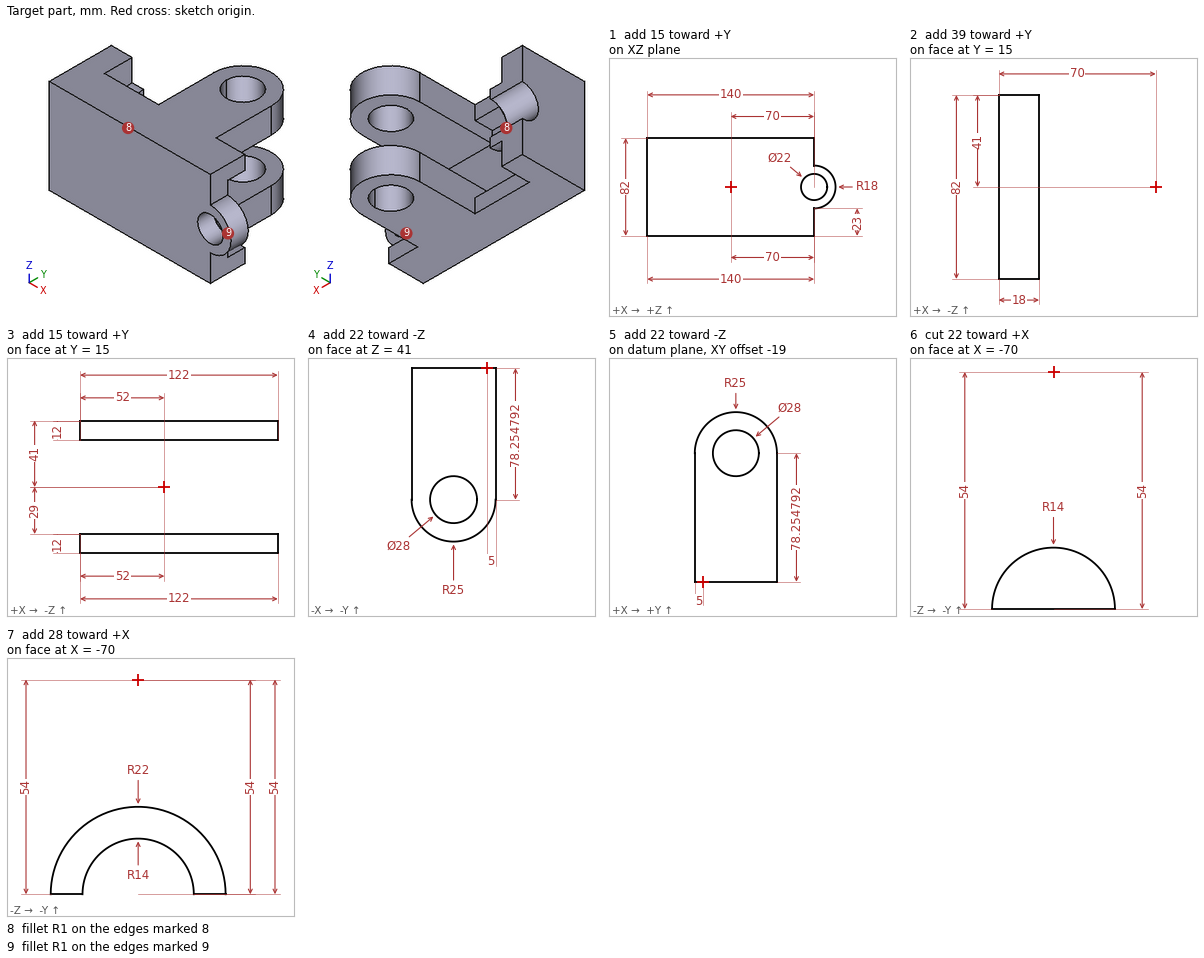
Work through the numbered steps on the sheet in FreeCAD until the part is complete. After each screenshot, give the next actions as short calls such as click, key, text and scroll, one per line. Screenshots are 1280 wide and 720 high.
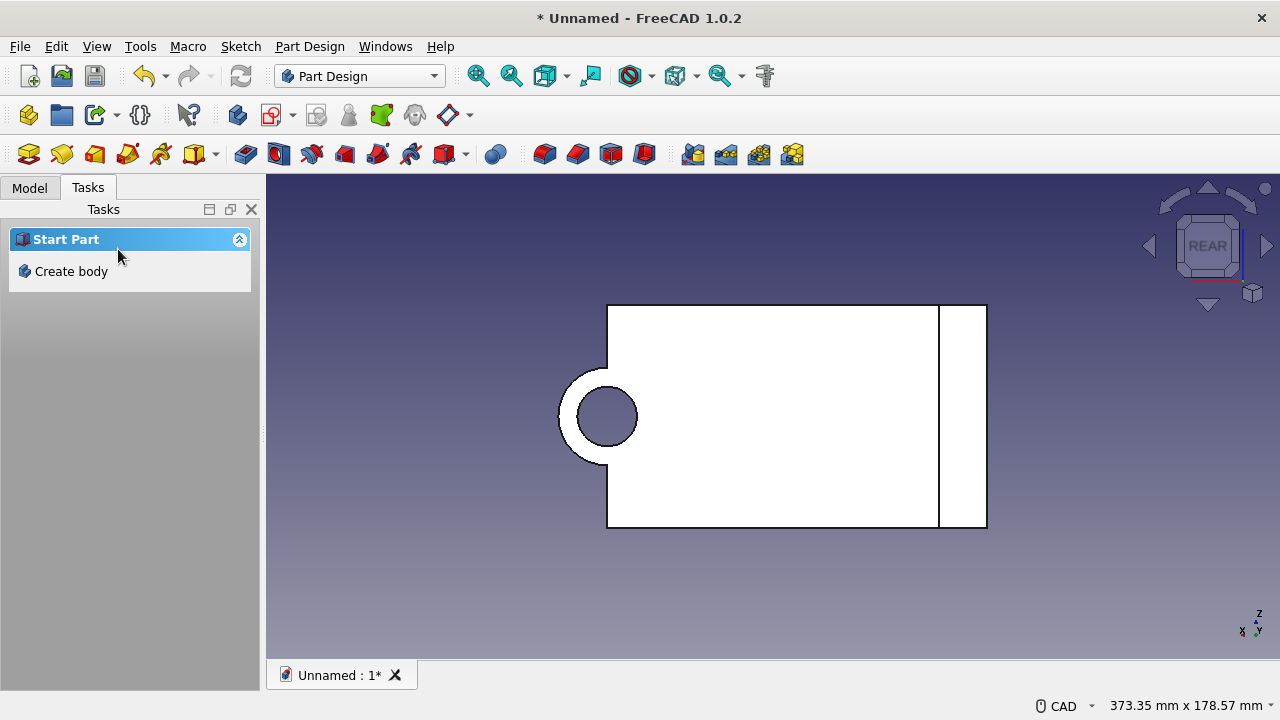
click(748, 416)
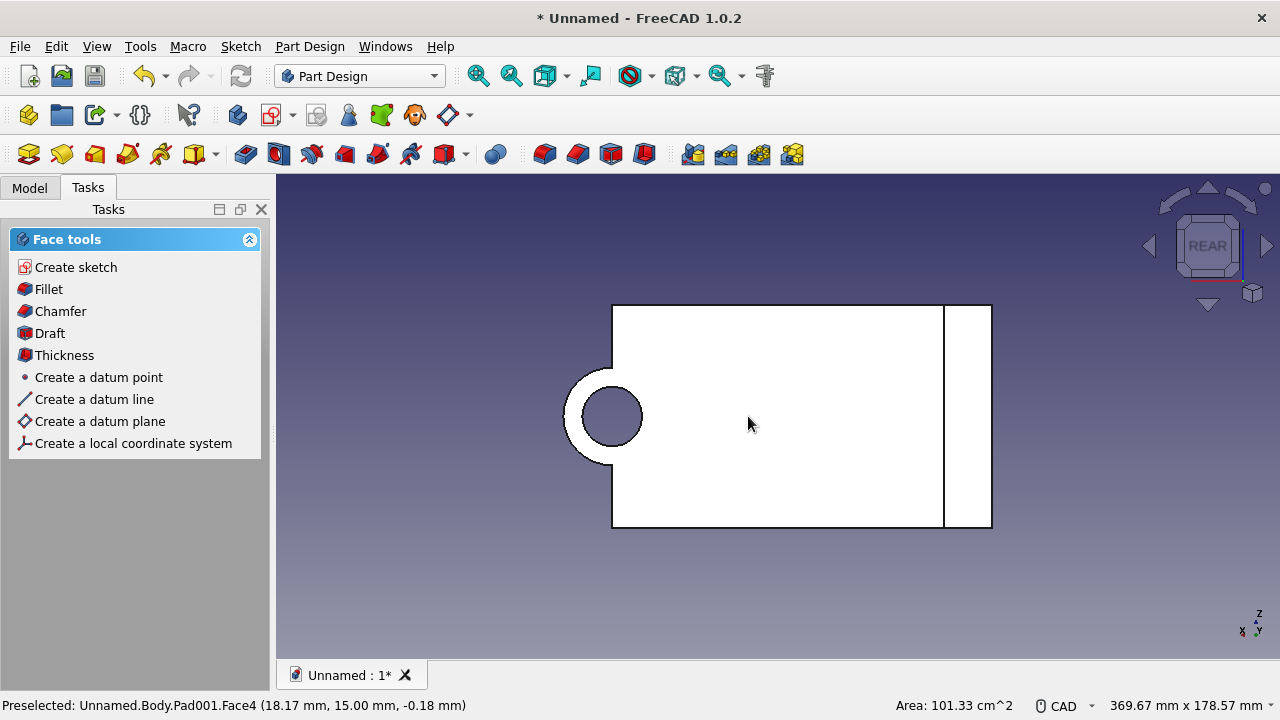
click(270, 116)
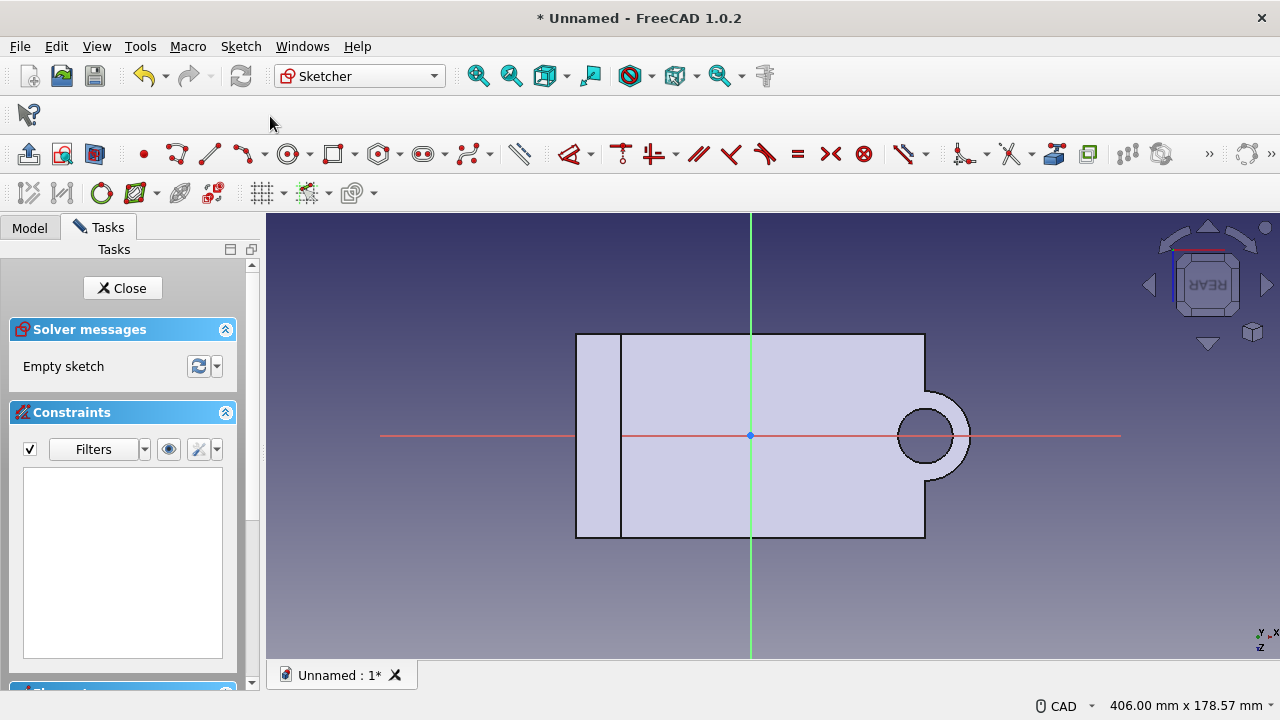
click(95, 154)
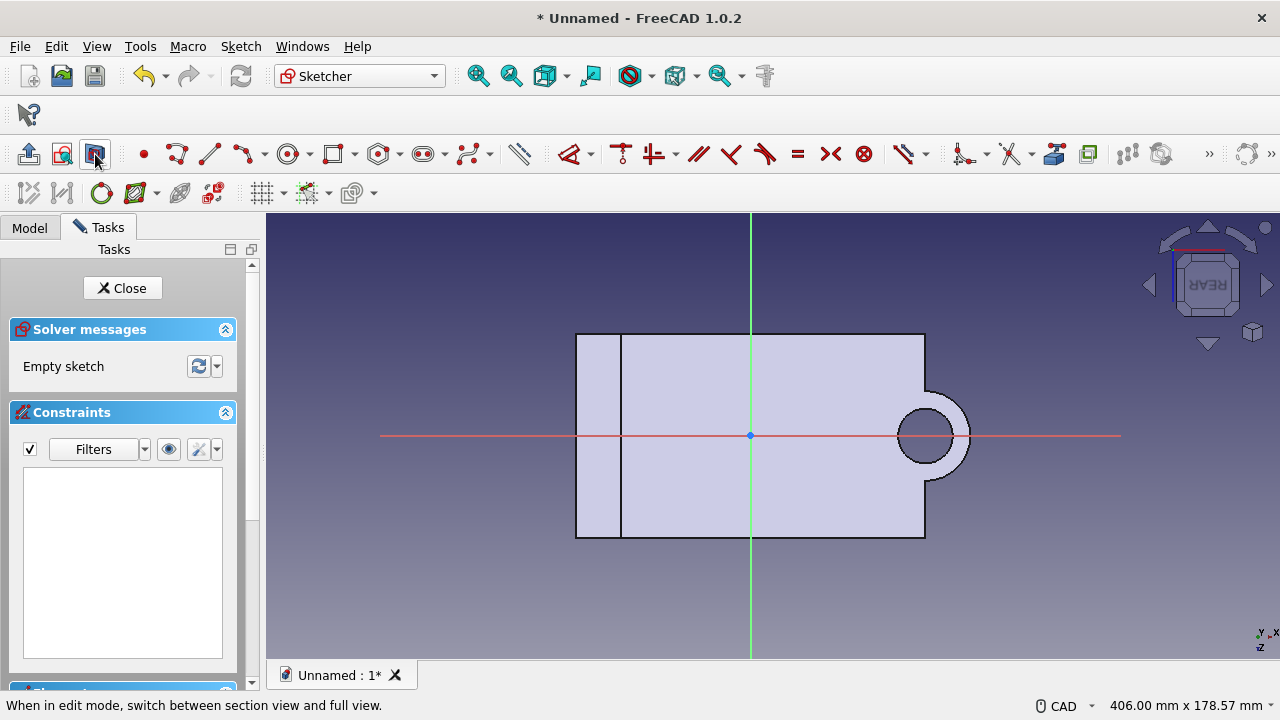
click(332, 154)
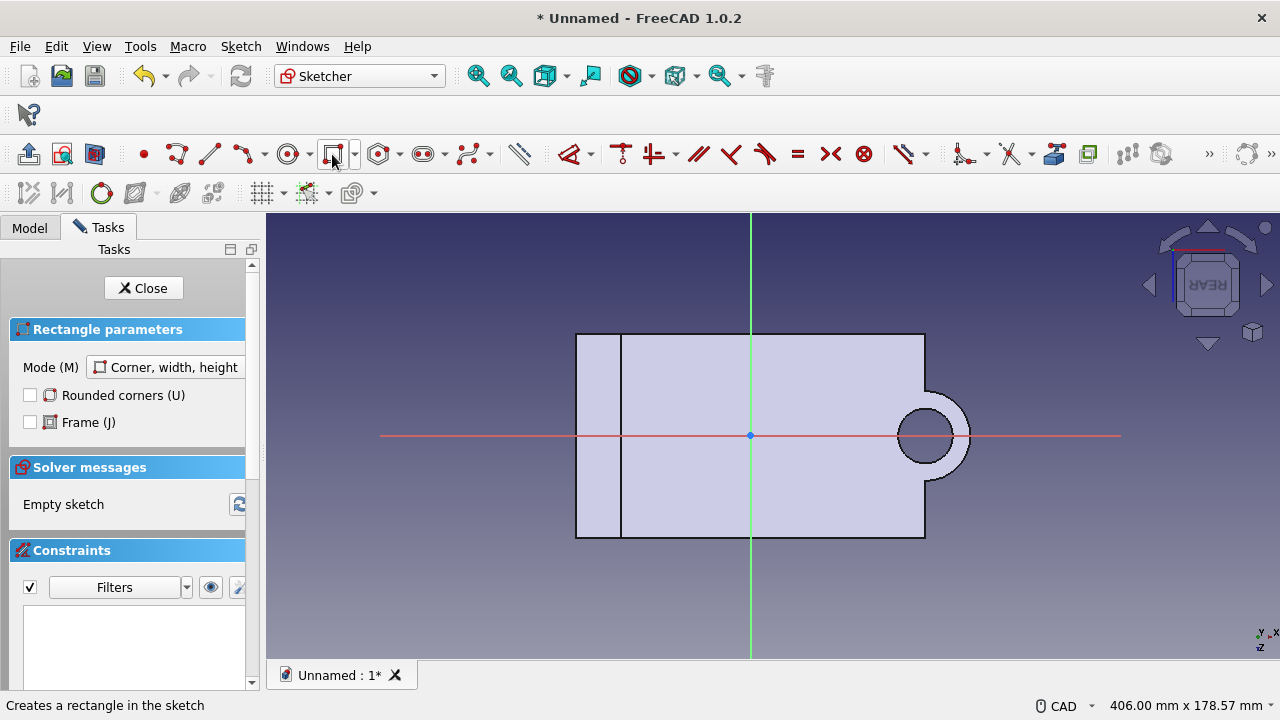
click(621, 334)
click(925, 364)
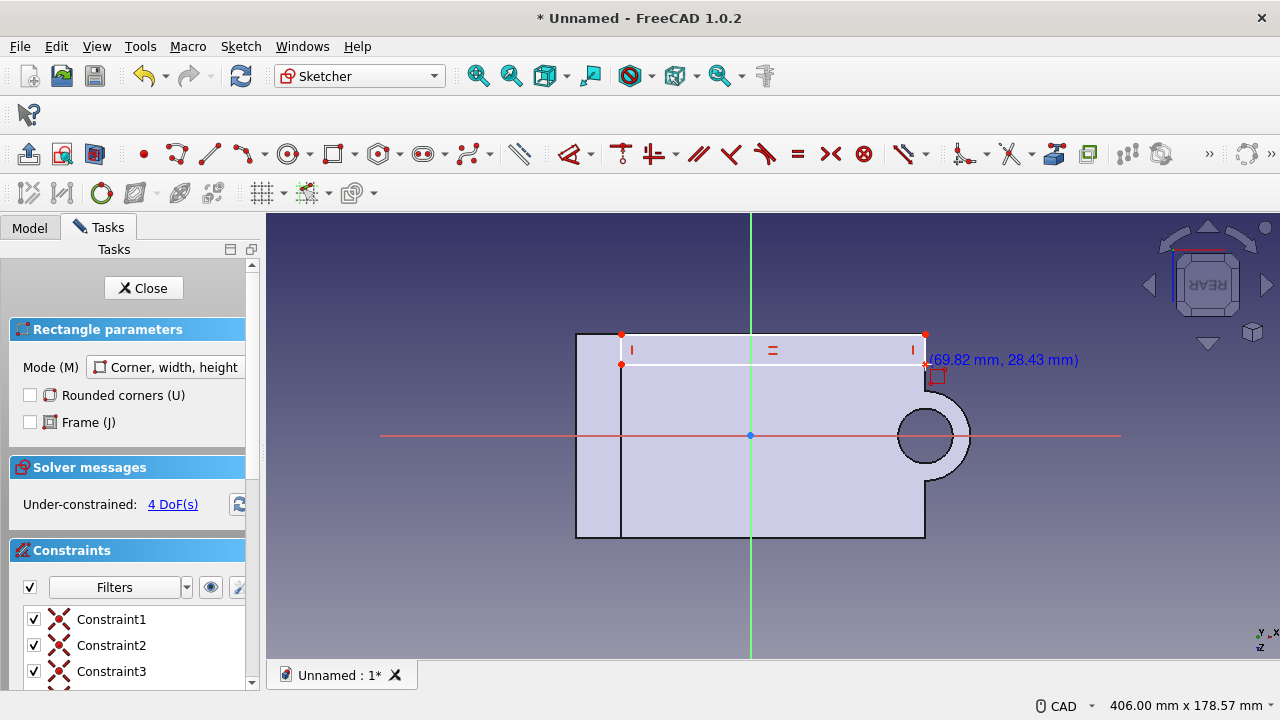
click(621, 508)
click(925, 538)
key(Escape)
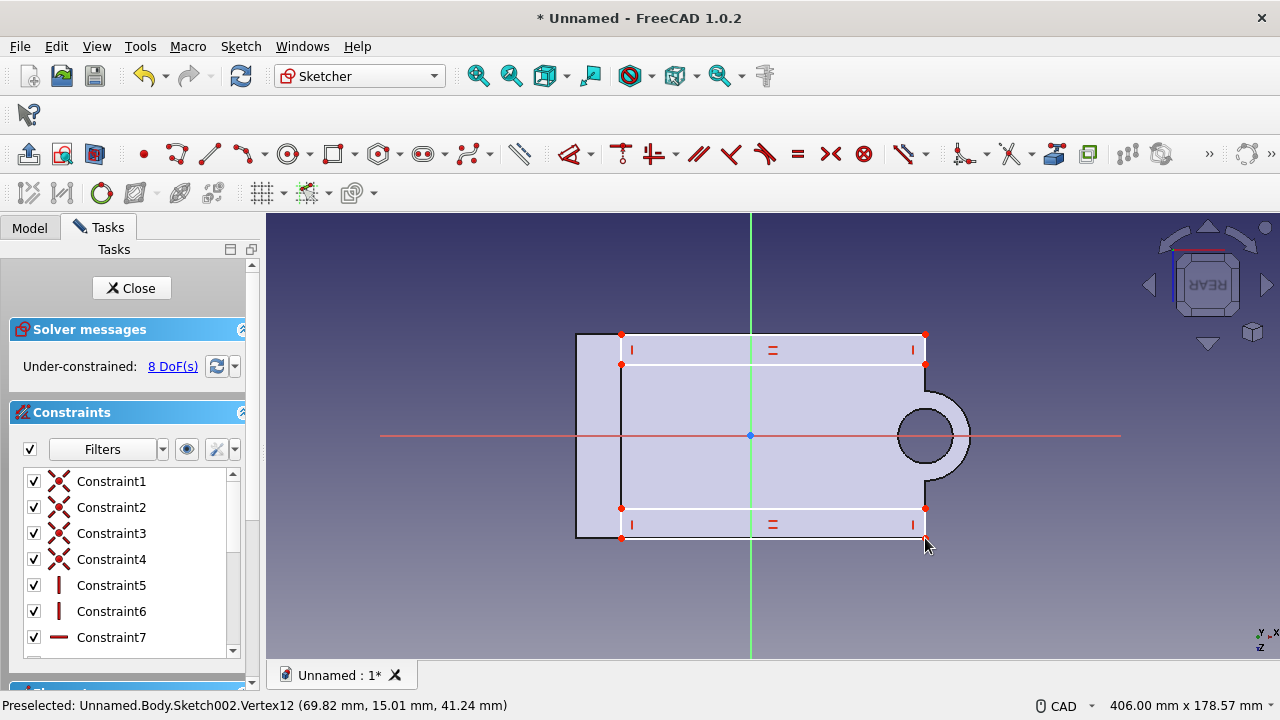
click(568, 154)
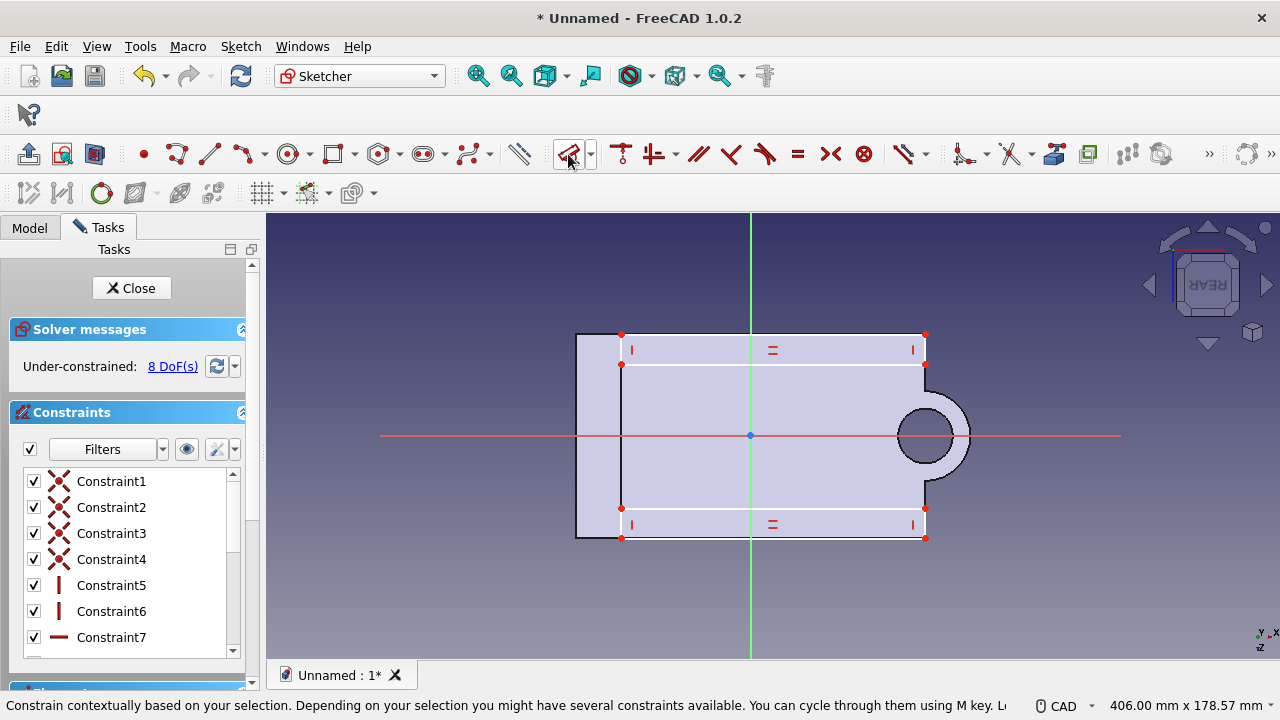
scroll(621, 344, up, 3)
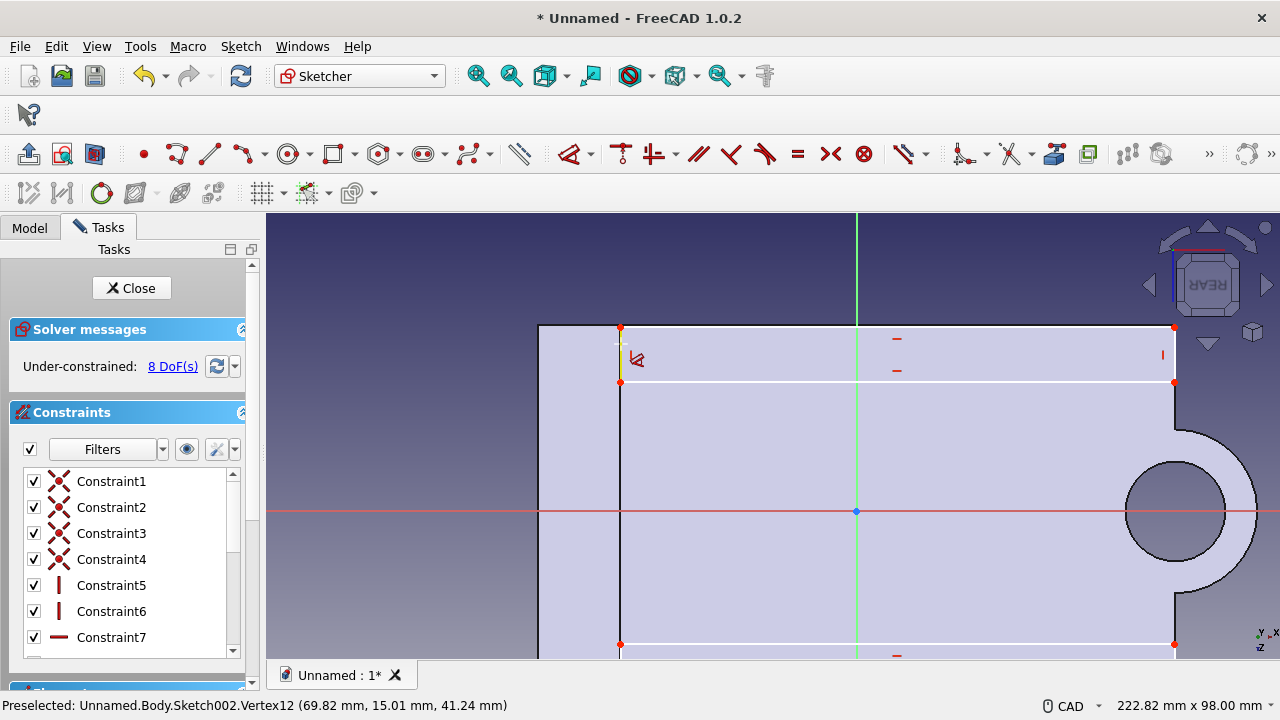
click(621, 344)
click(587, 355)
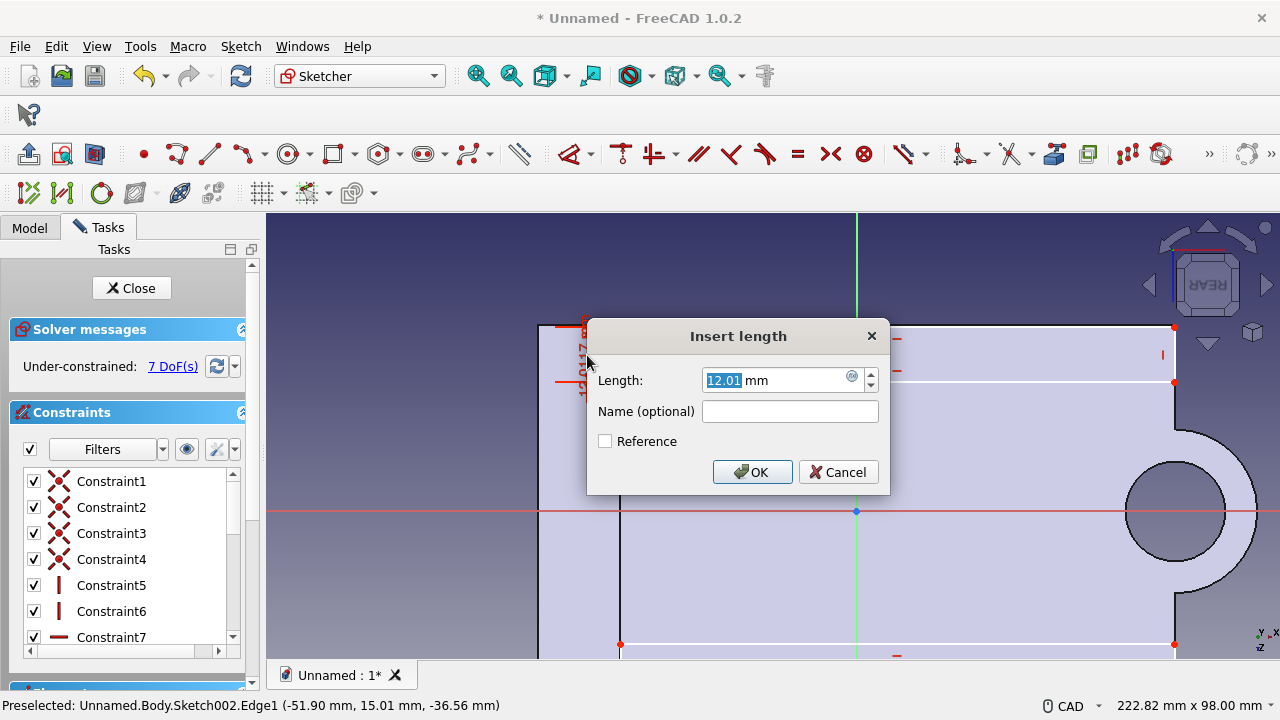
text(12)
key(Return)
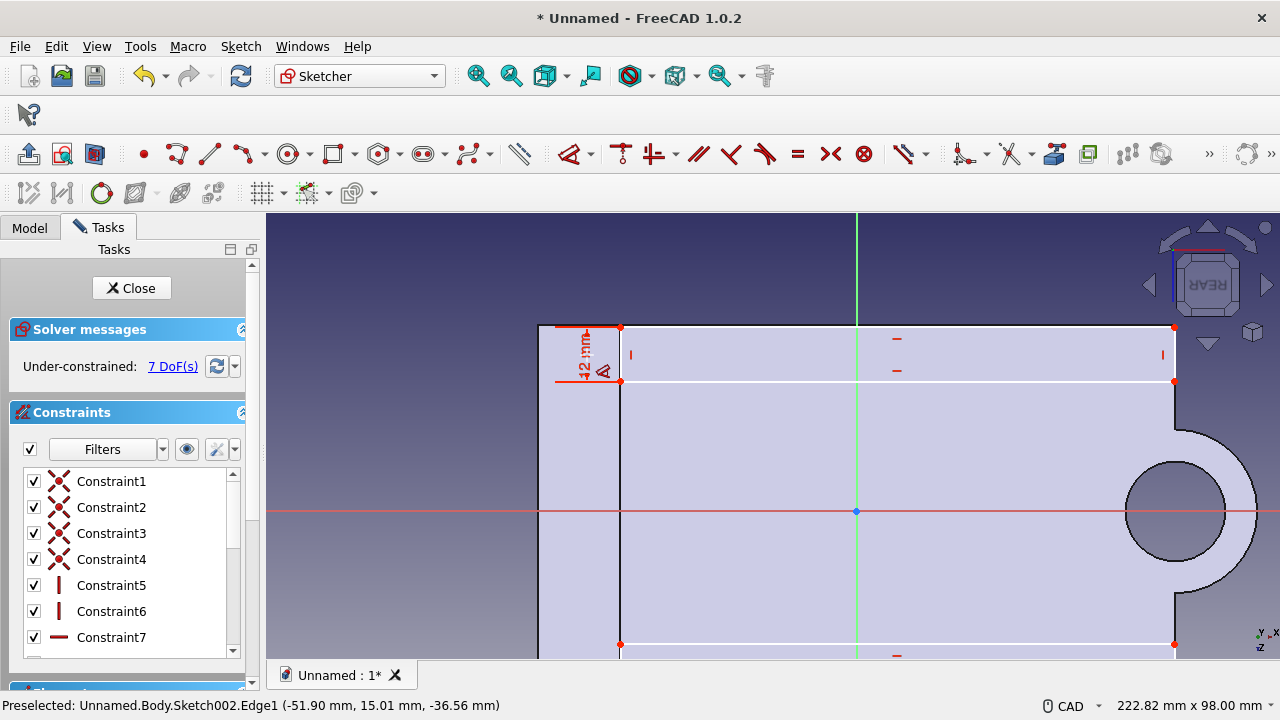
scroll(311, 283, down, 2)